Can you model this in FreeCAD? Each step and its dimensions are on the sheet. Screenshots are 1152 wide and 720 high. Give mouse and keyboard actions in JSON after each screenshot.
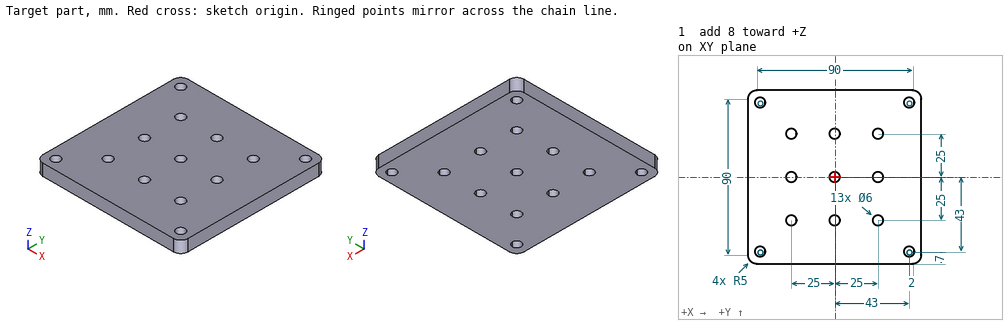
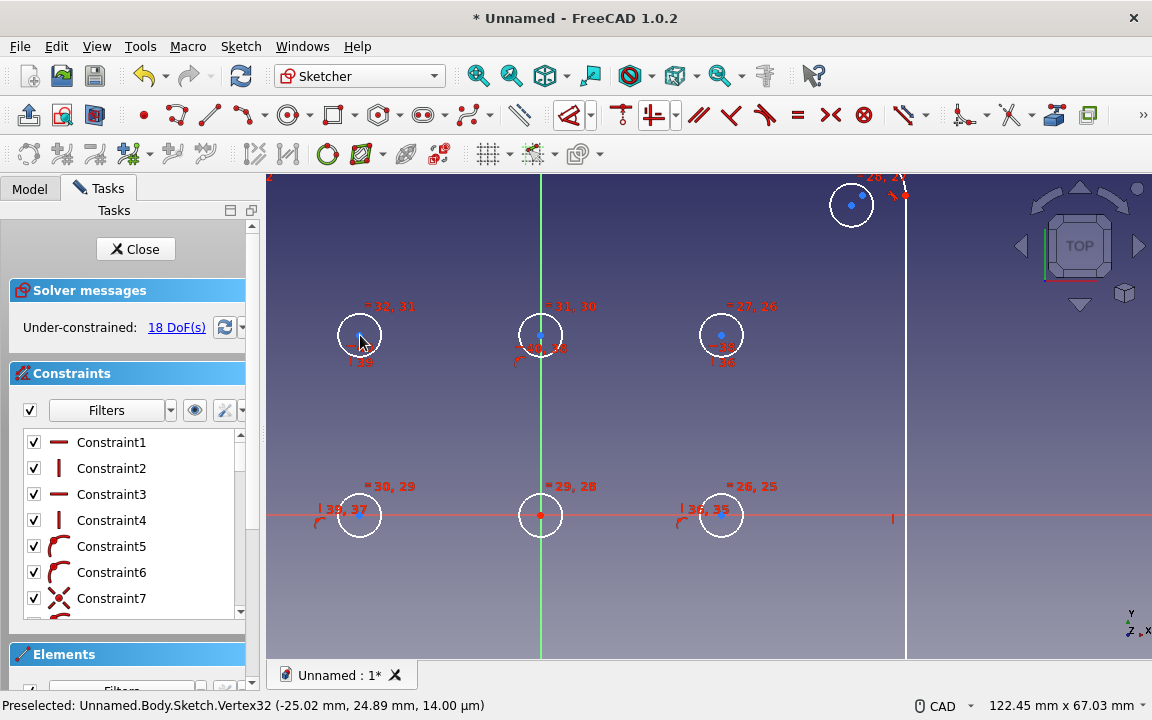
{"action": "scroll", "coordinate": [722, 336], "scroll_direction": "down", "scroll_amount": 4}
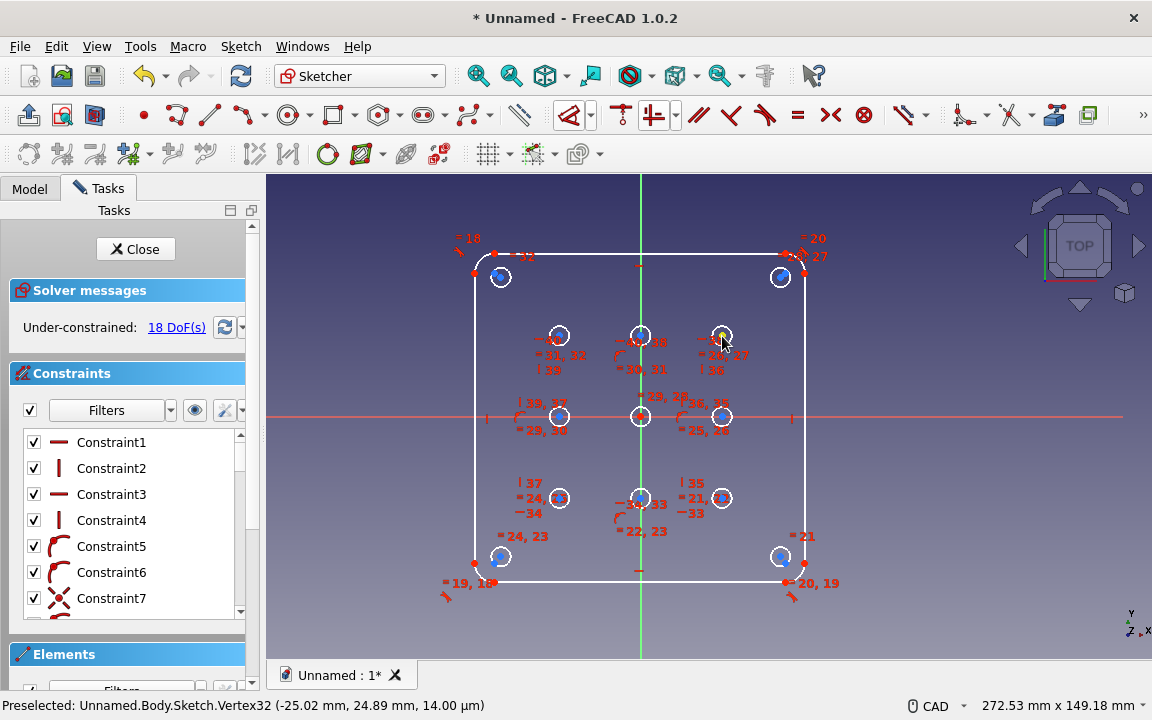
{"action": "scroll", "coordinate": [781, 557], "scroll_direction": "up", "scroll_amount": 3}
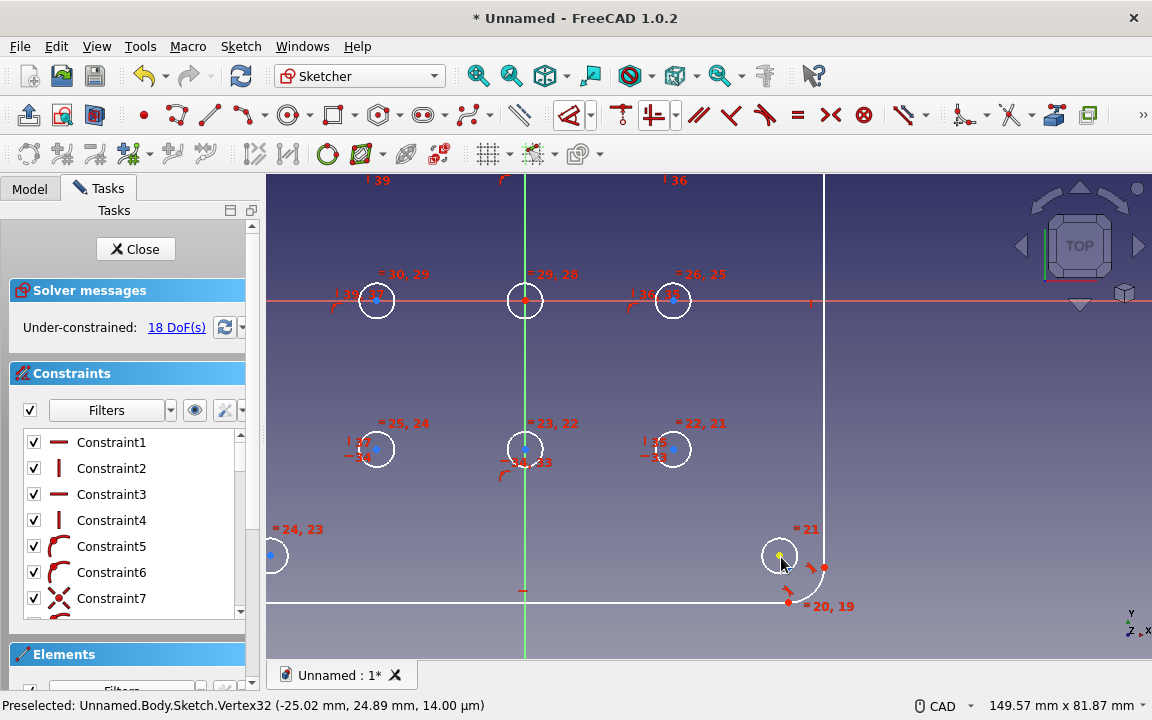
{"action": "left_click", "coordinate": [780, 556]}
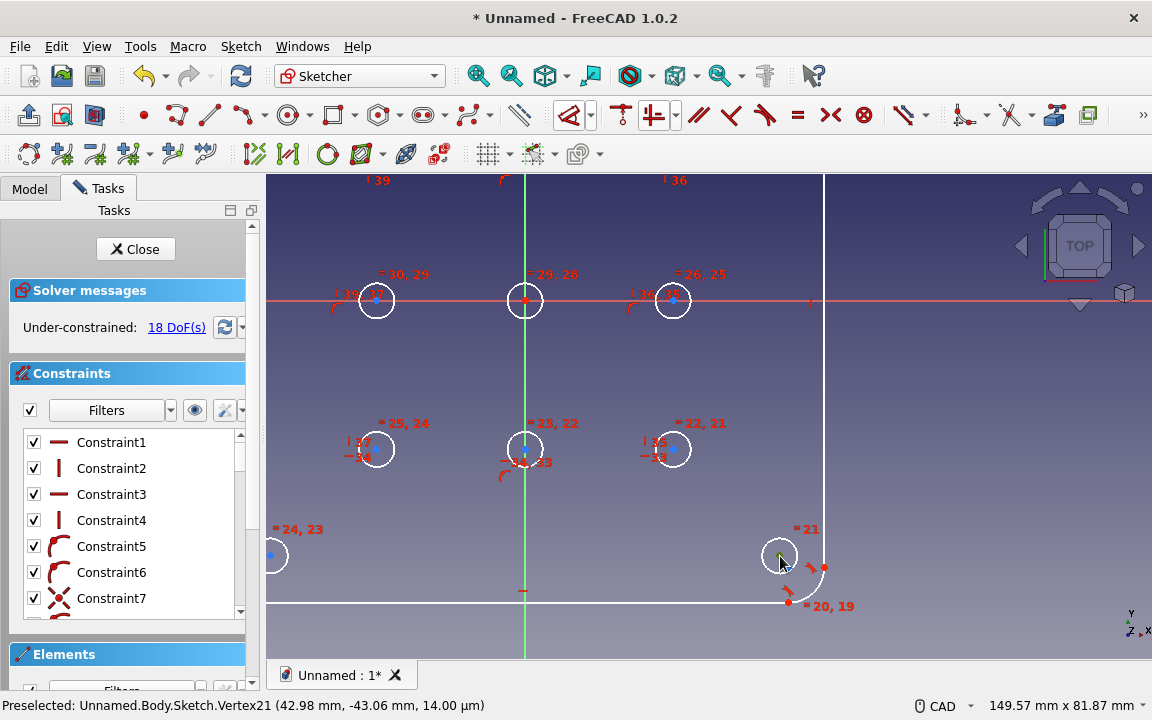
{"action": "scroll", "coordinate": [781, 557], "scroll_direction": "down", "scroll_amount": 3}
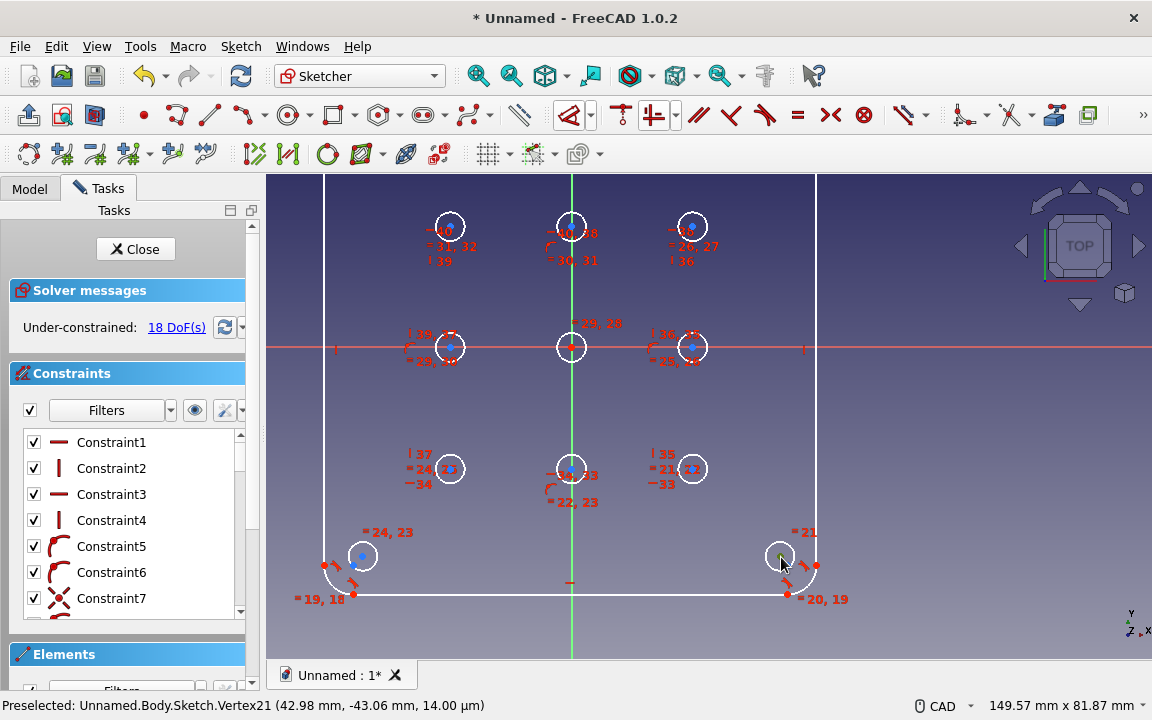
{"action": "scroll", "coordinate": [501, 557], "scroll_direction": "up", "scroll_amount": 2}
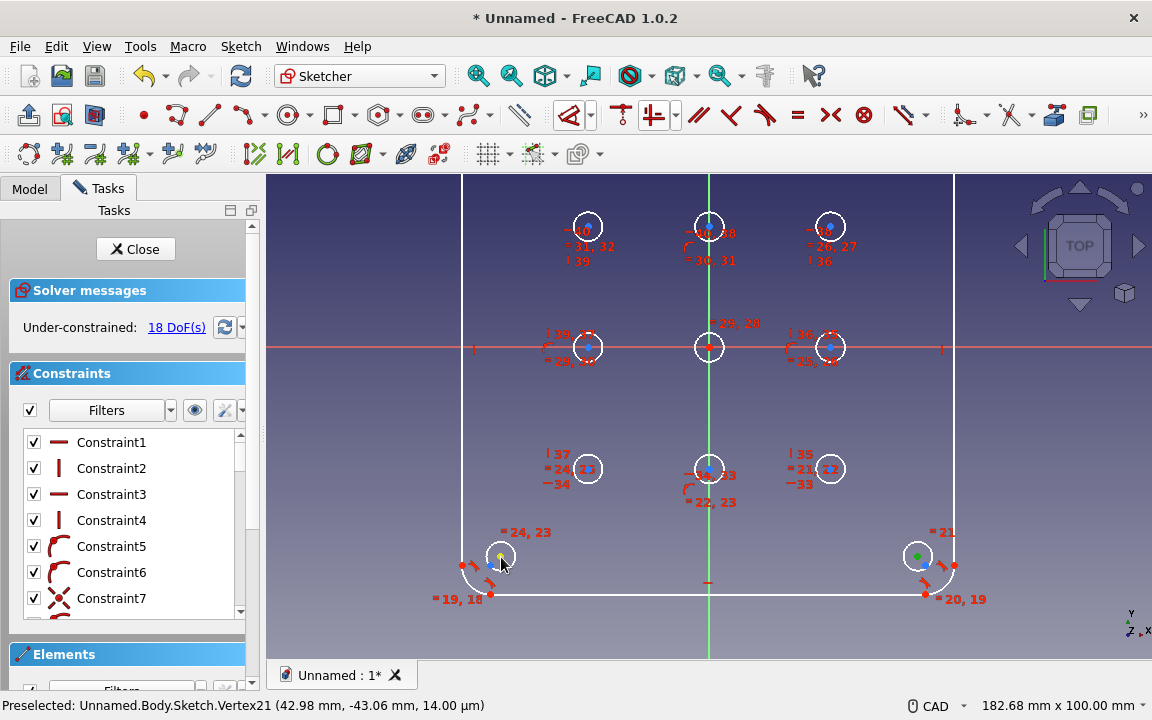
{"action": "left_click", "coordinate": [501, 556]}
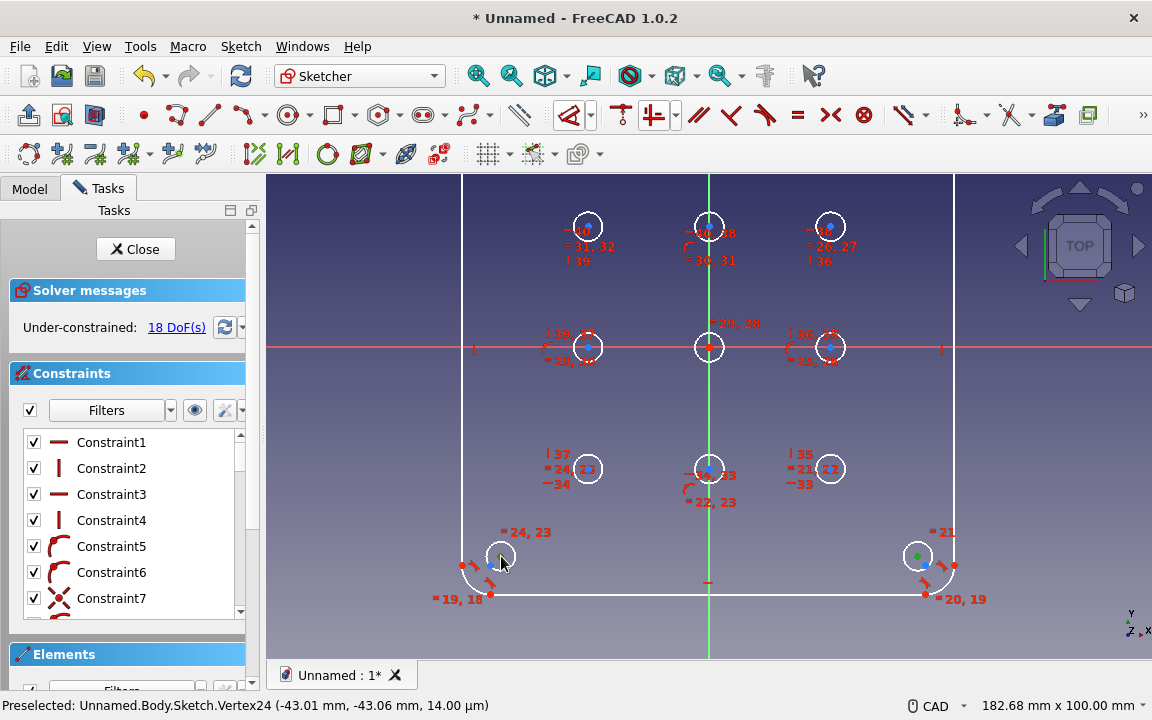
{"action": "left_click", "coordinate": [709, 539]}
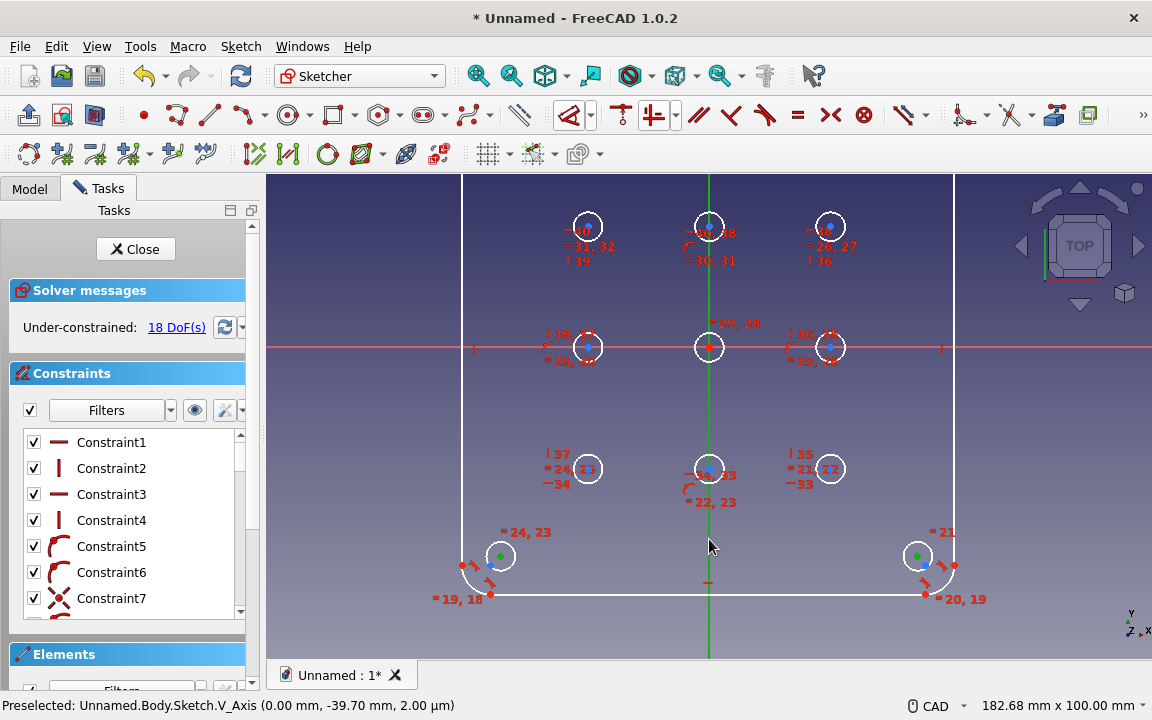
{"action": "left_click", "coordinate": [831, 116]}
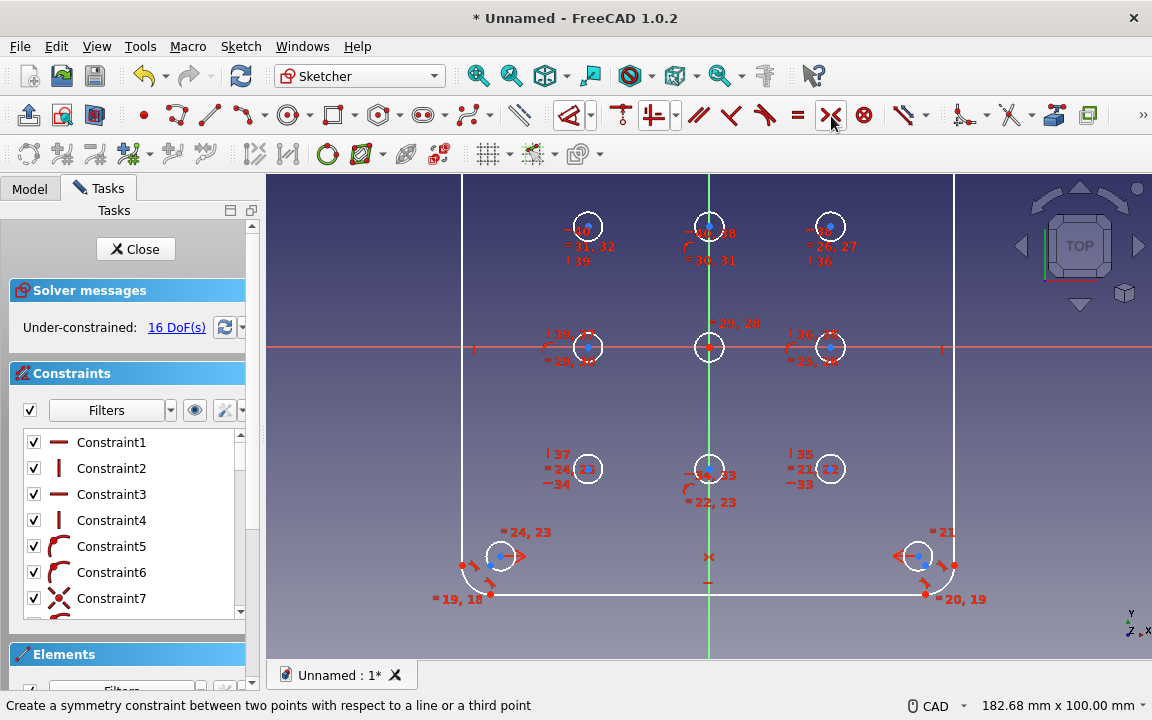
{"action": "left_click", "coordinate": [918, 556]}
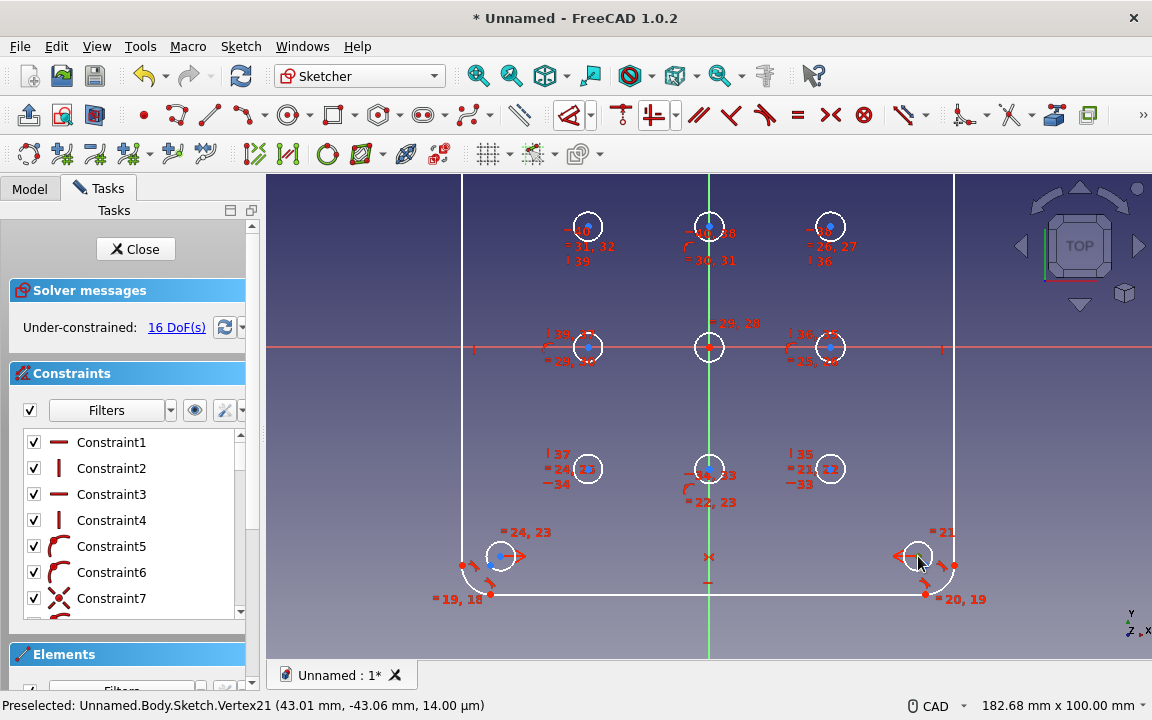
{"action": "scroll", "coordinate": [500, 557], "scroll_direction": "down", "scroll_amount": 2}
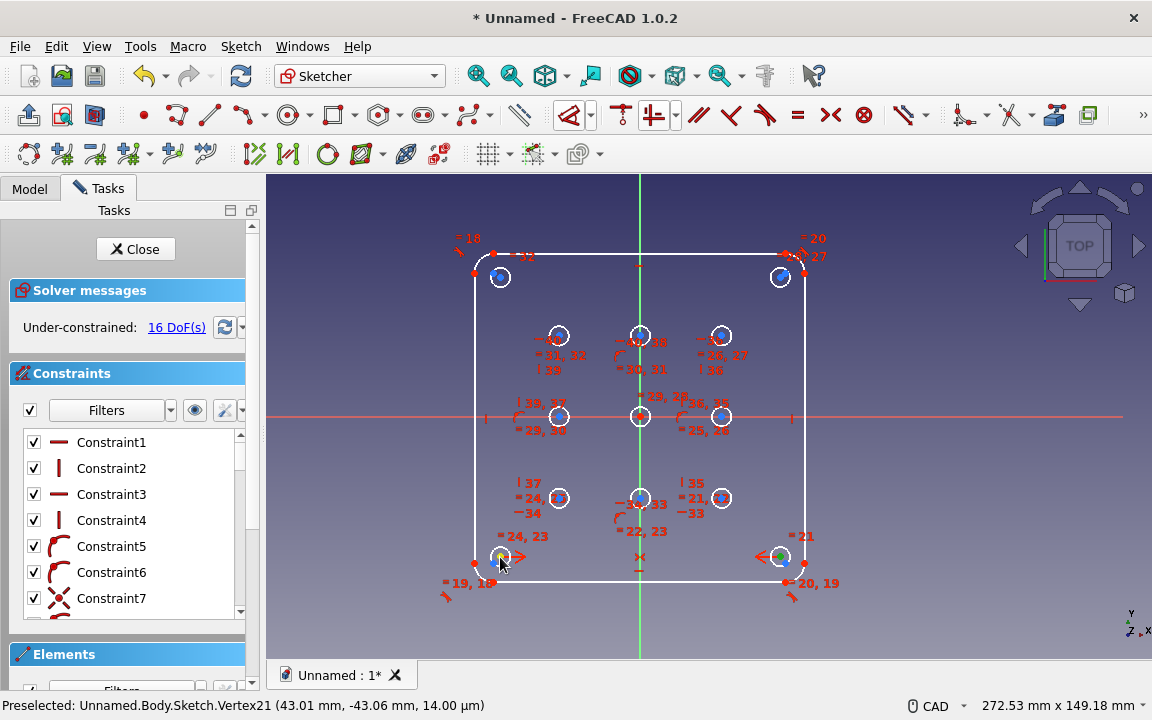
{"action": "scroll", "coordinate": [780, 277], "scroll_direction": "up", "scroll_amount": 4}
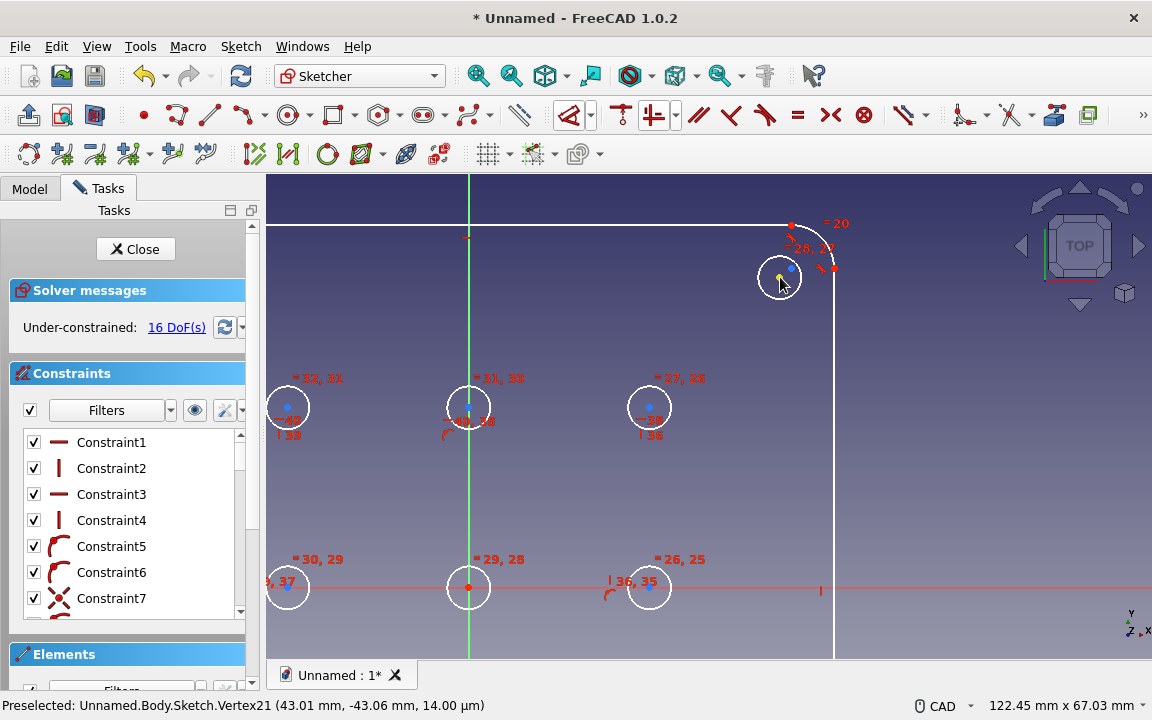
{"action": "left_click", "coordinate": [780, 278]}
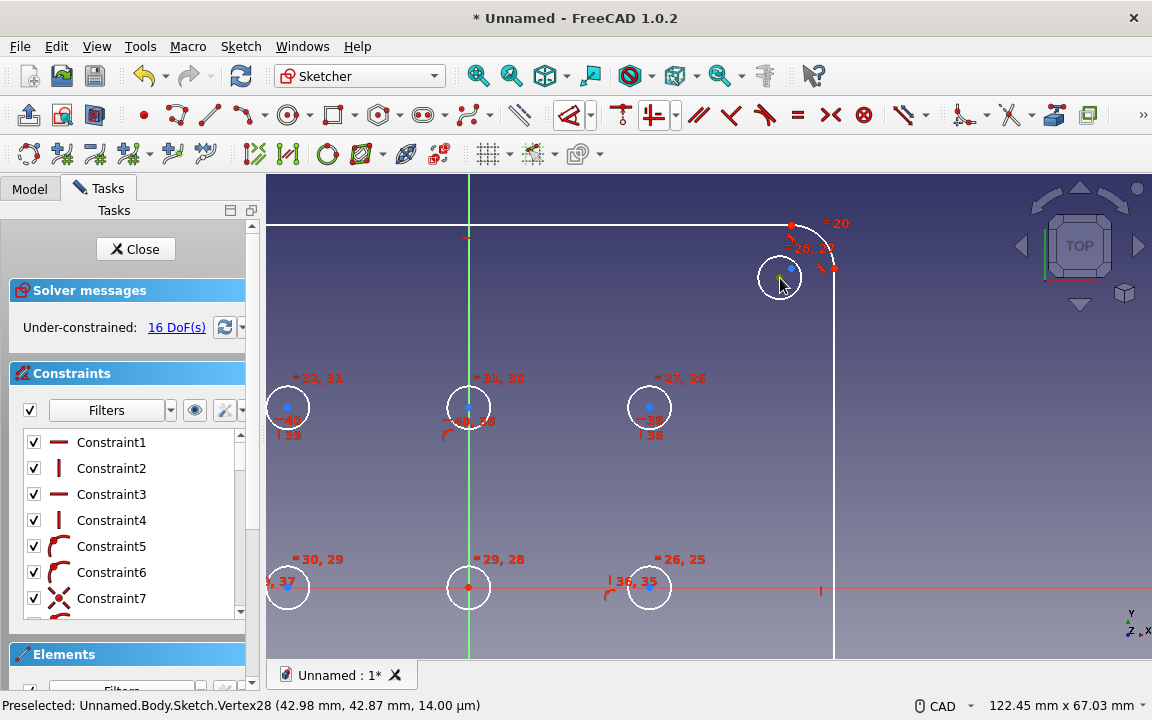
{"action": "left_click", "coordinate": [344, 588]}